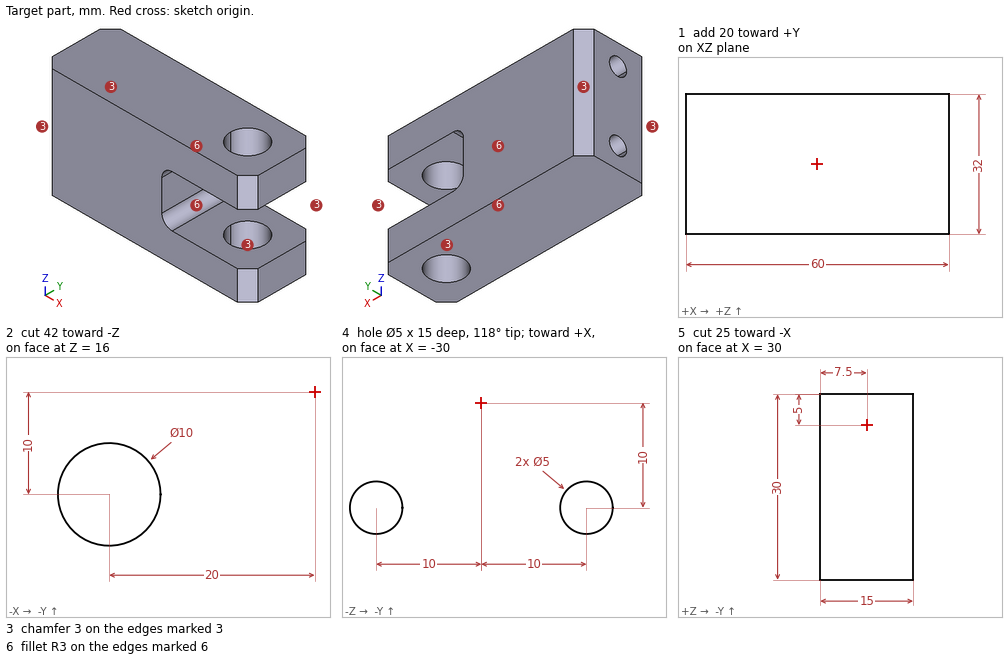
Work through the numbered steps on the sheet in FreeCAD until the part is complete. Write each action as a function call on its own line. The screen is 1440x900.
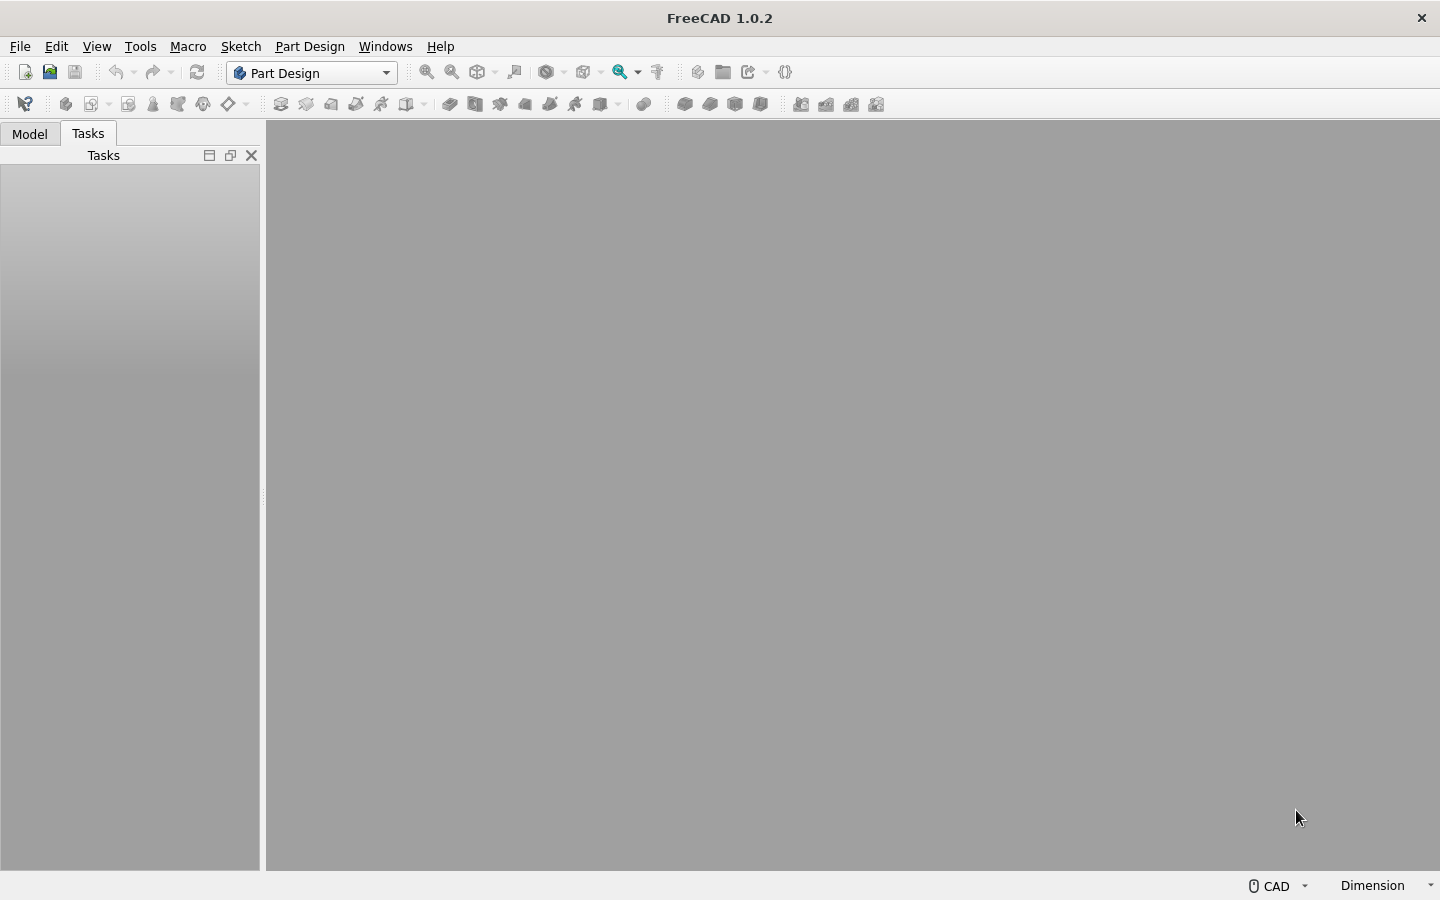
click(25, 72)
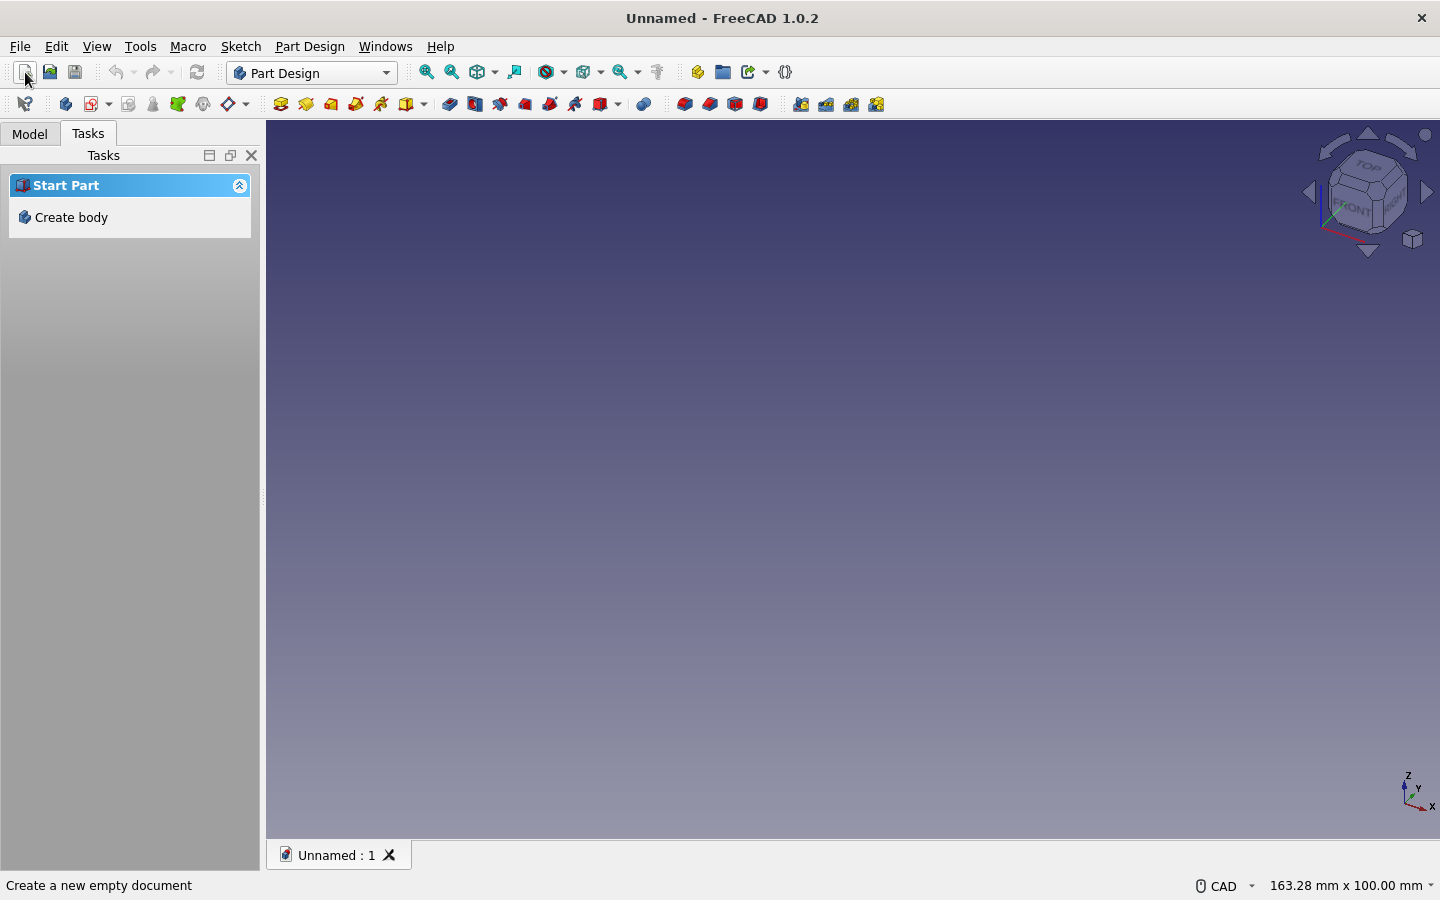
click(90, 104)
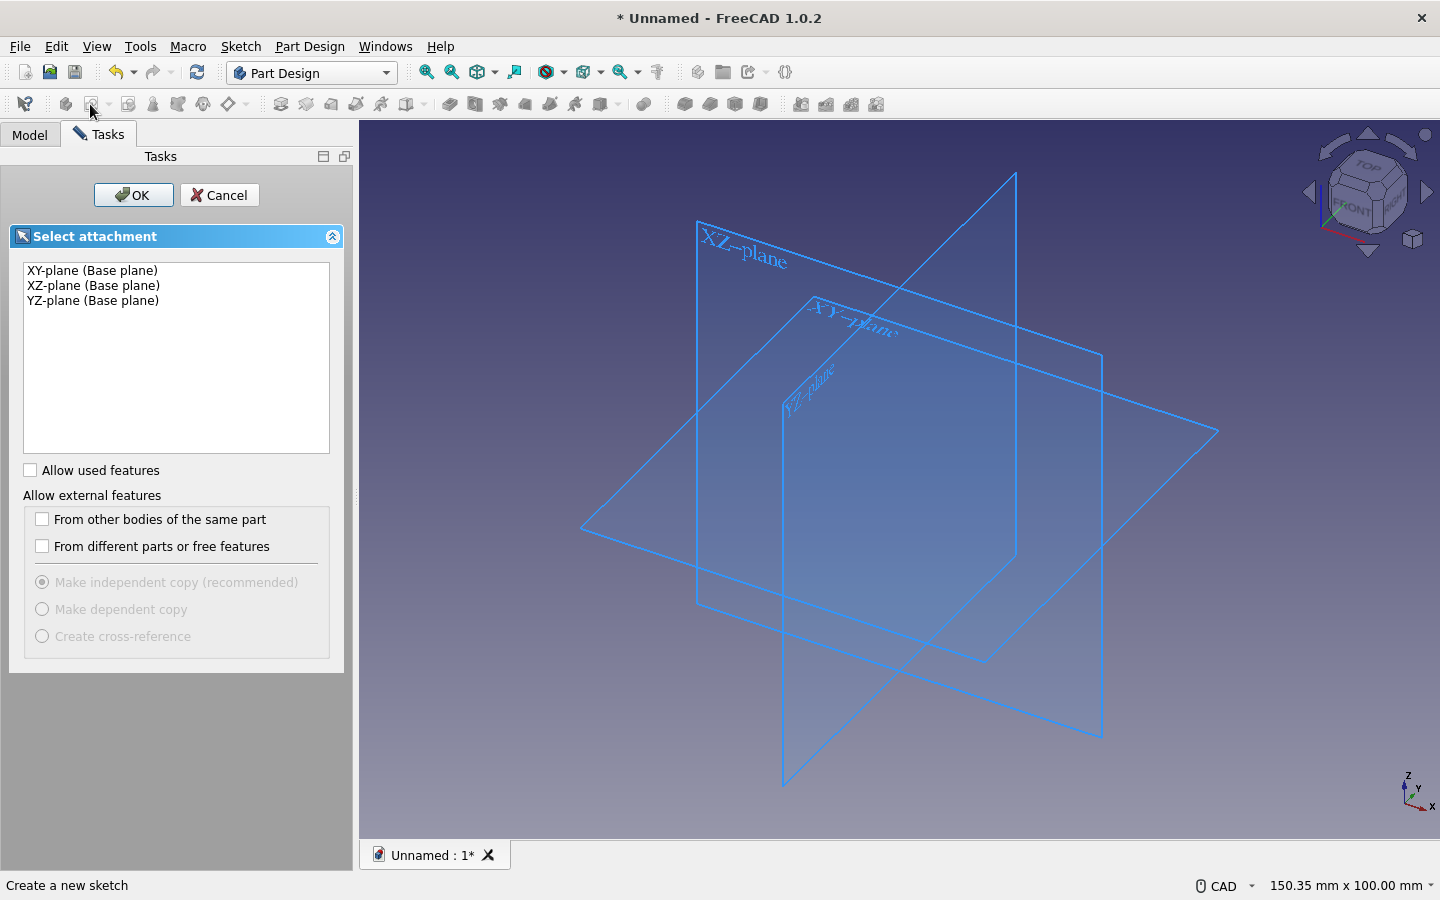
click(84, 286)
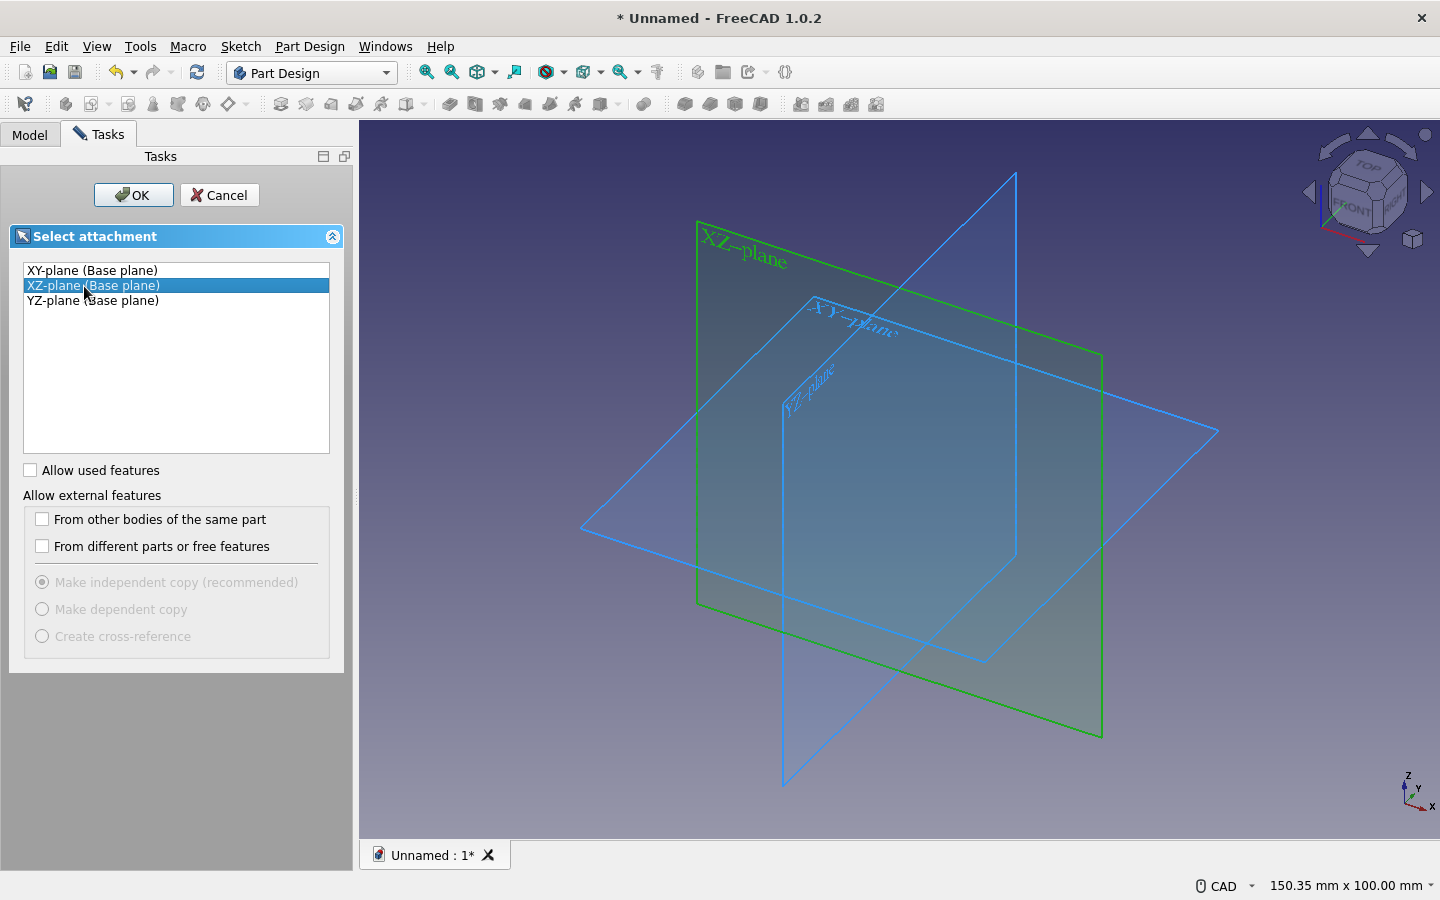
click(134, 195)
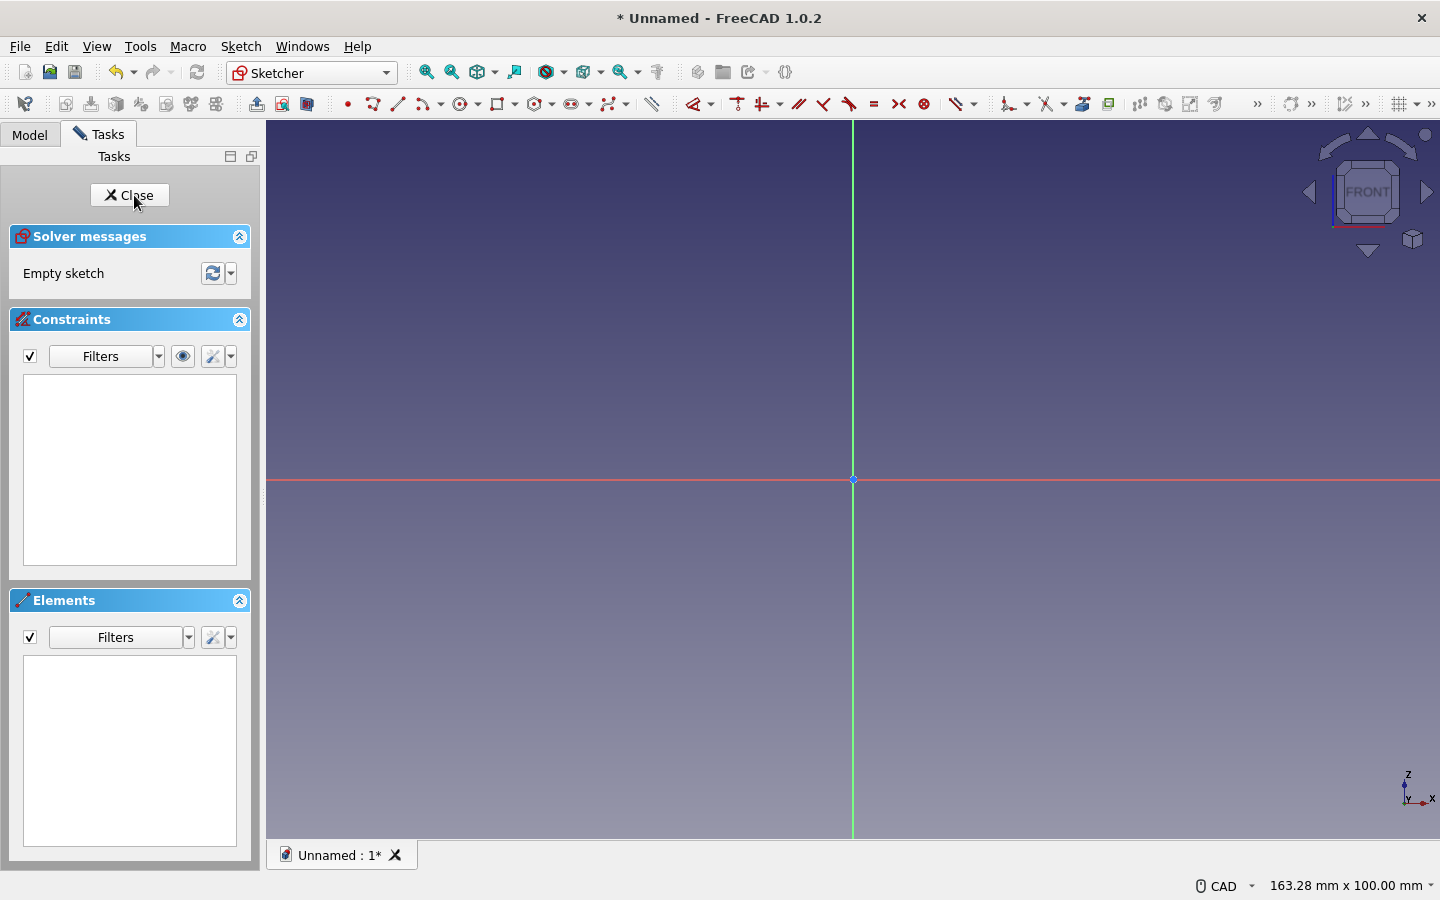
scroll(992, 480, up, 2)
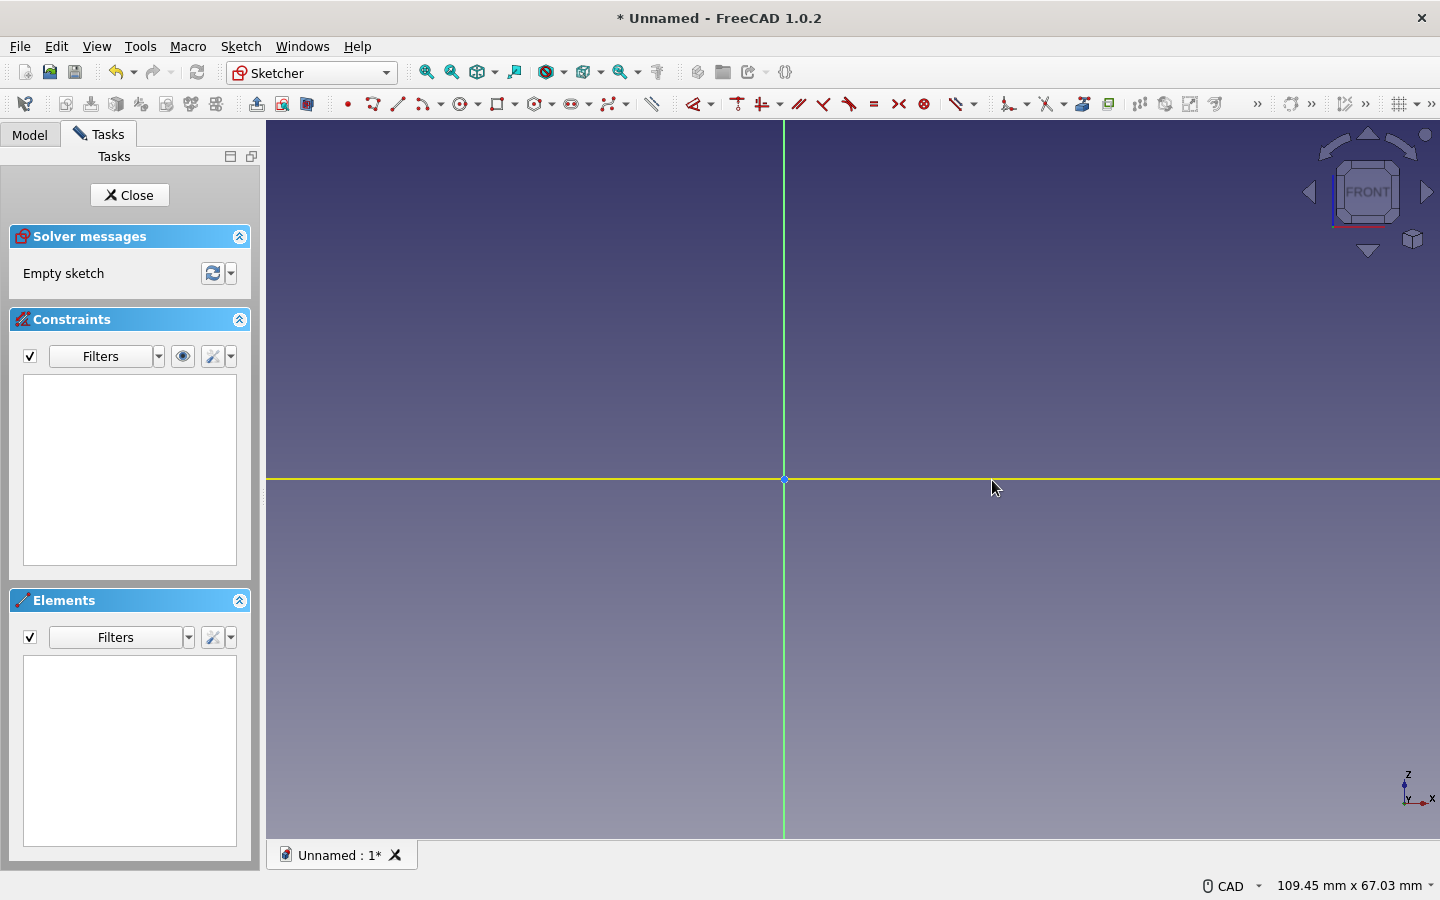
click(514, 104)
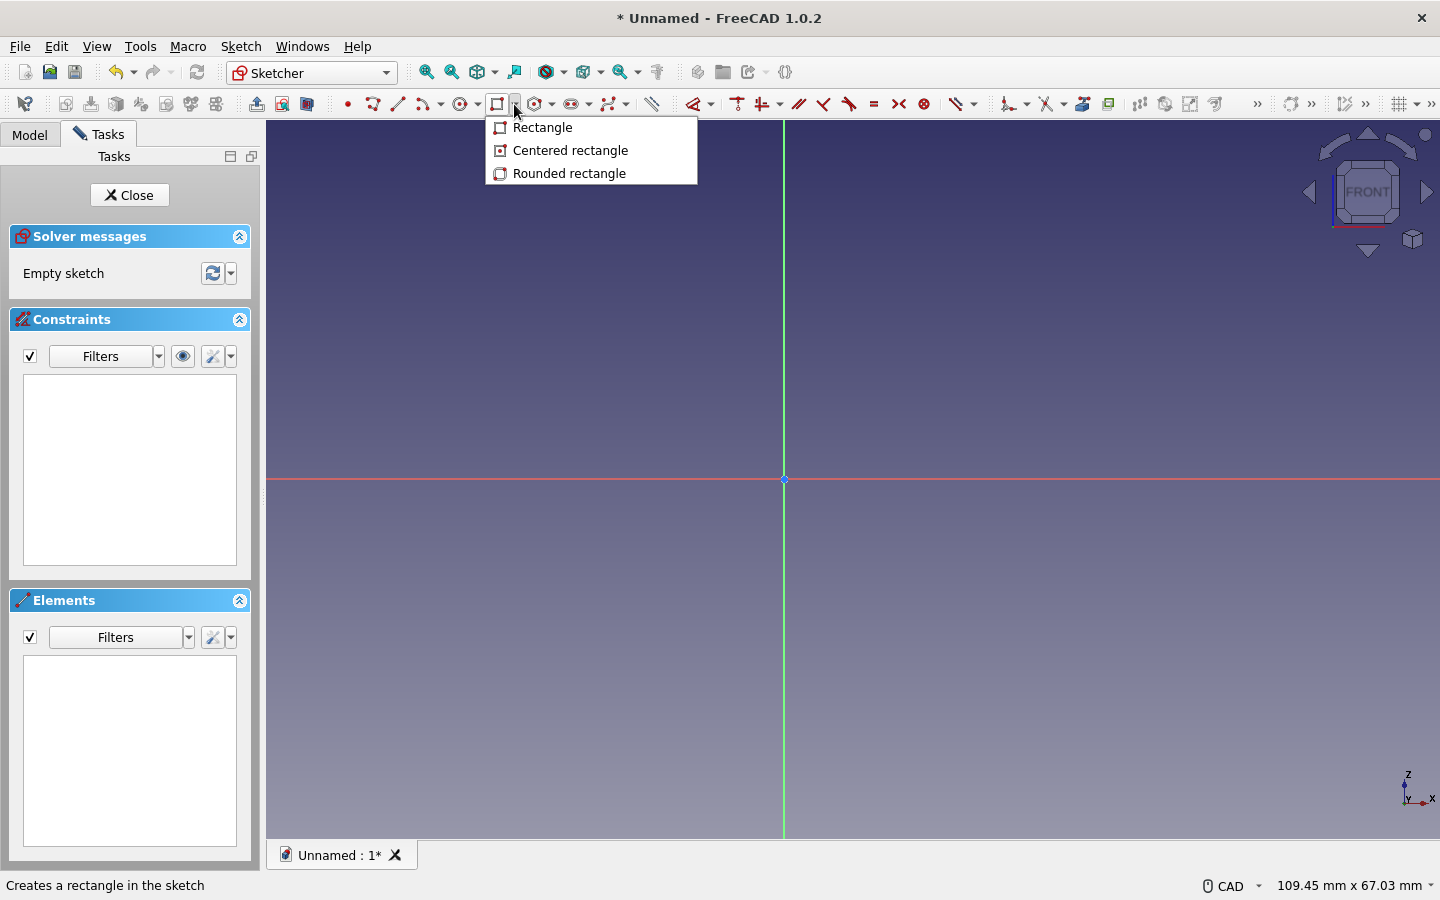
click(592, 150)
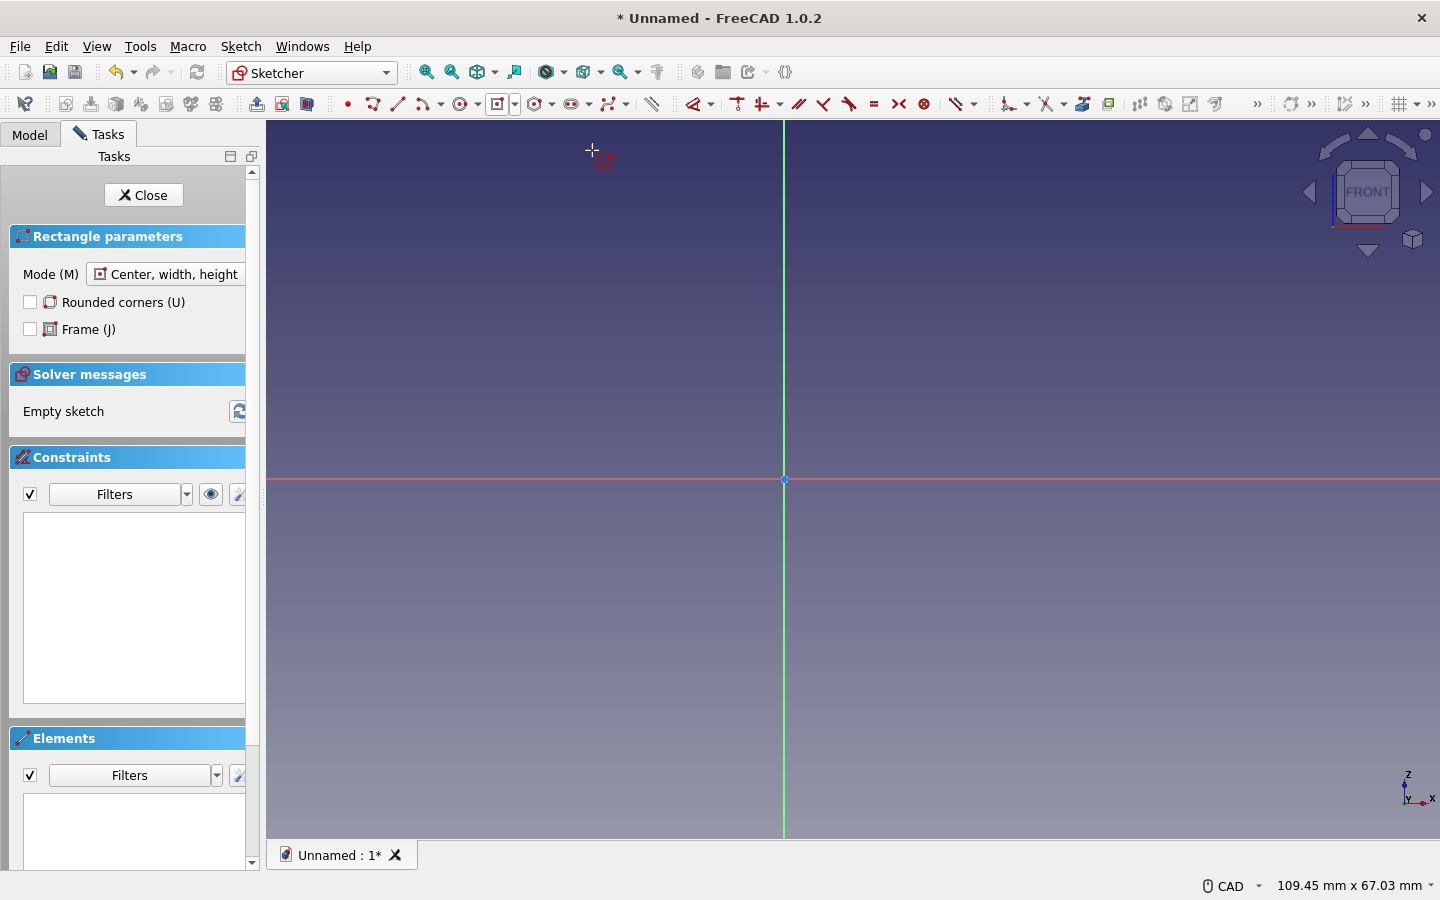
click(784, 479)
click(1106, 307)
key(Escape)